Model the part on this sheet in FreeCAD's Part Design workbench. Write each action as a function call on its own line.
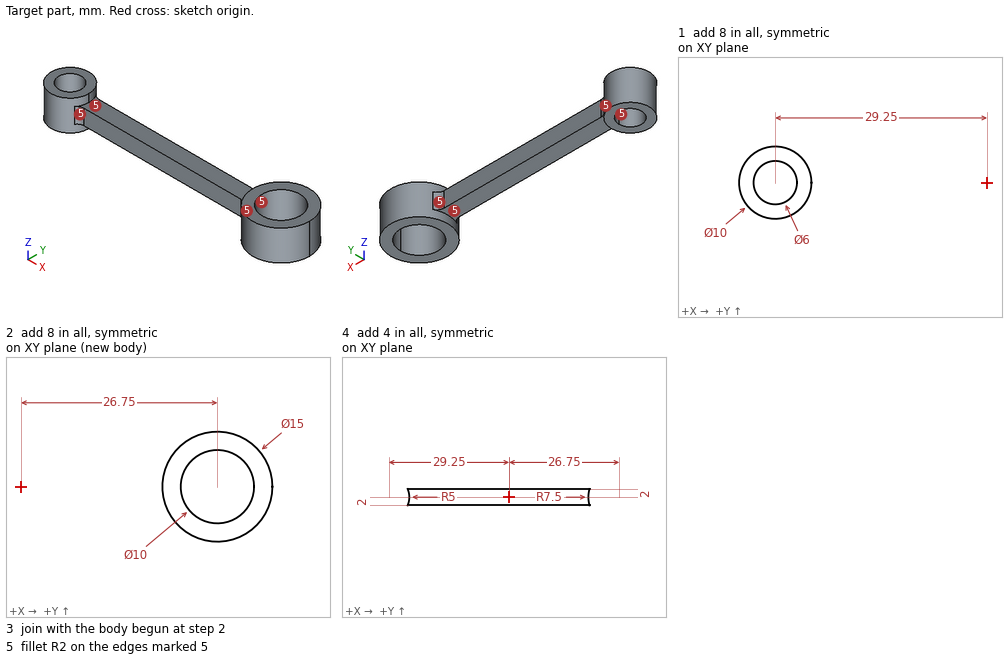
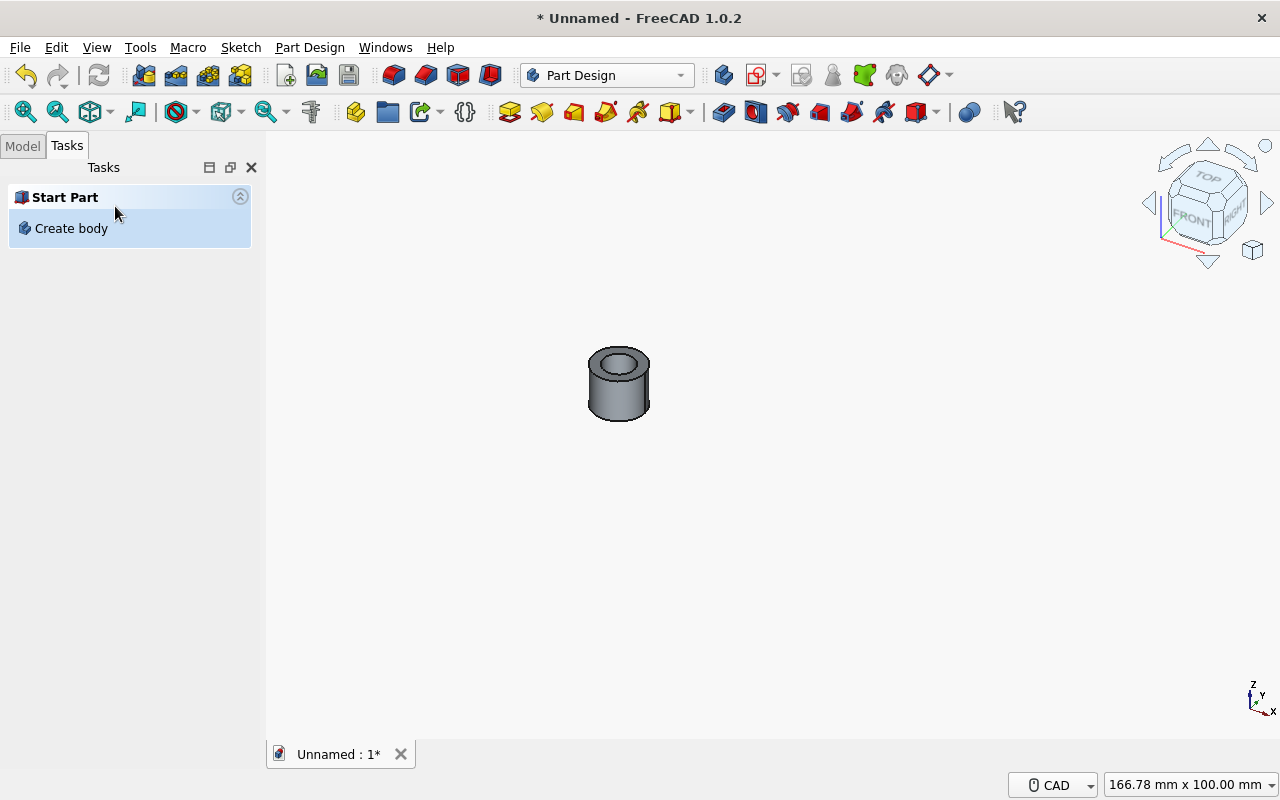
click(26, 112)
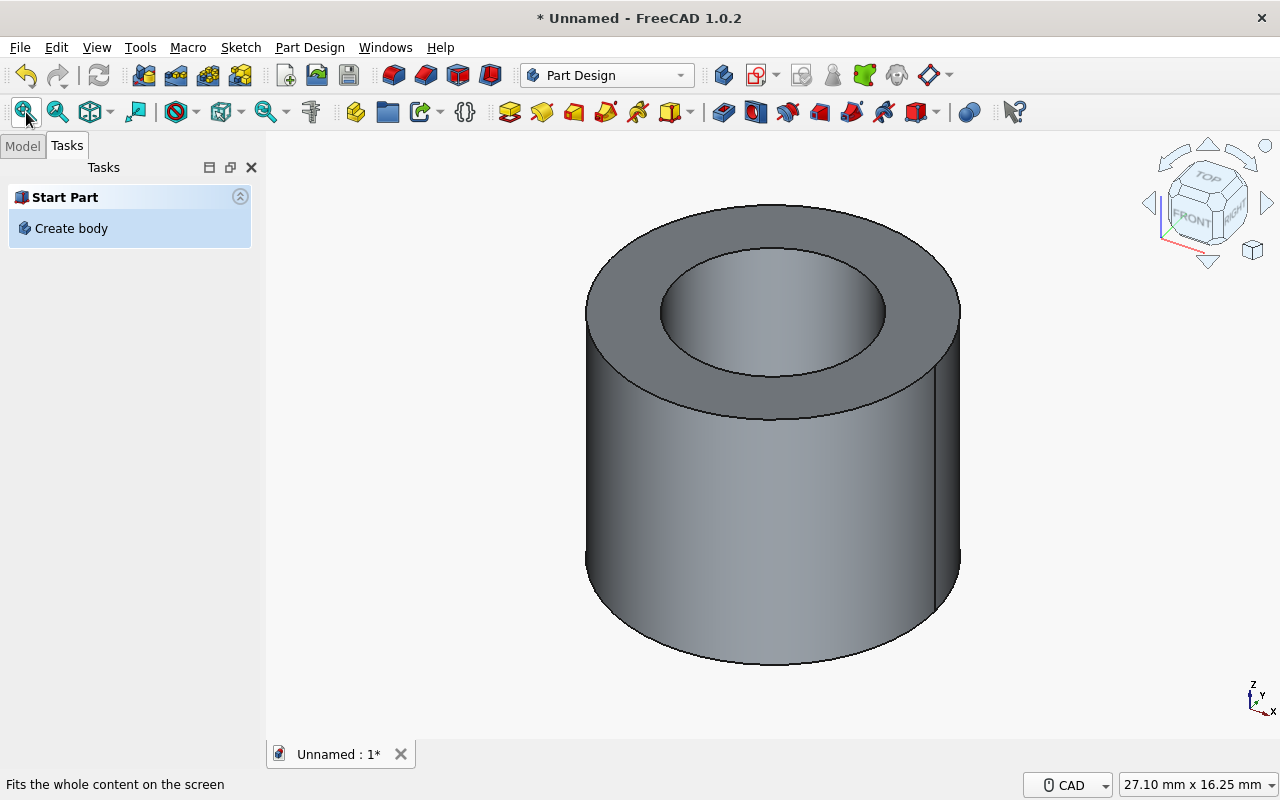
click(724, 76)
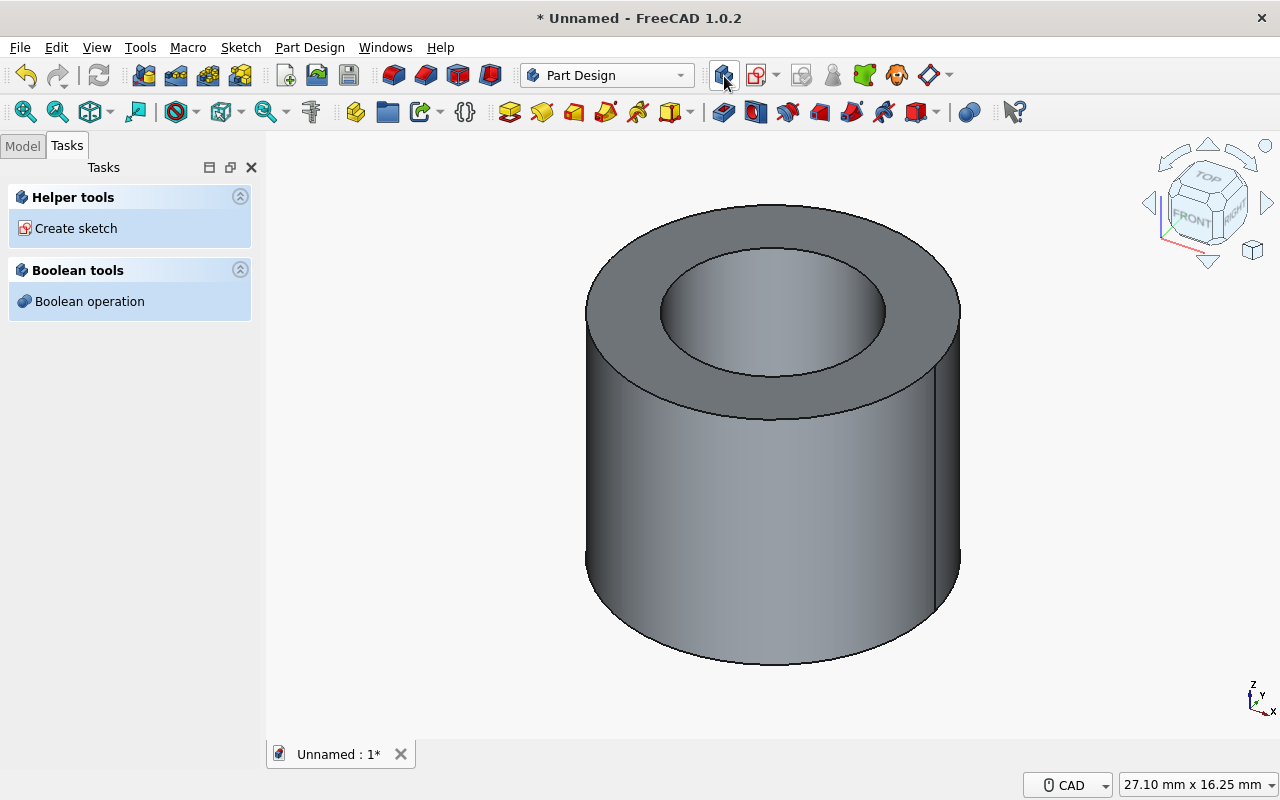
click(306, 699)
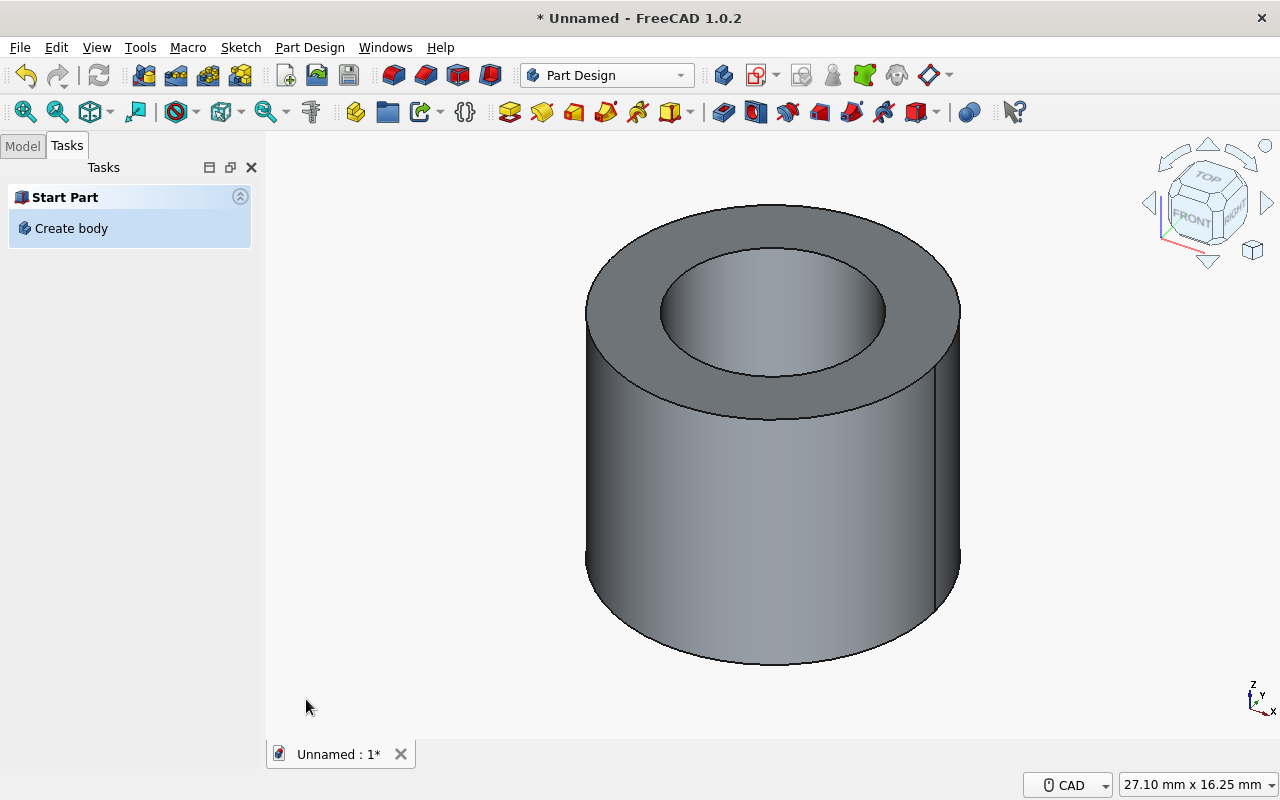
click(756, 76)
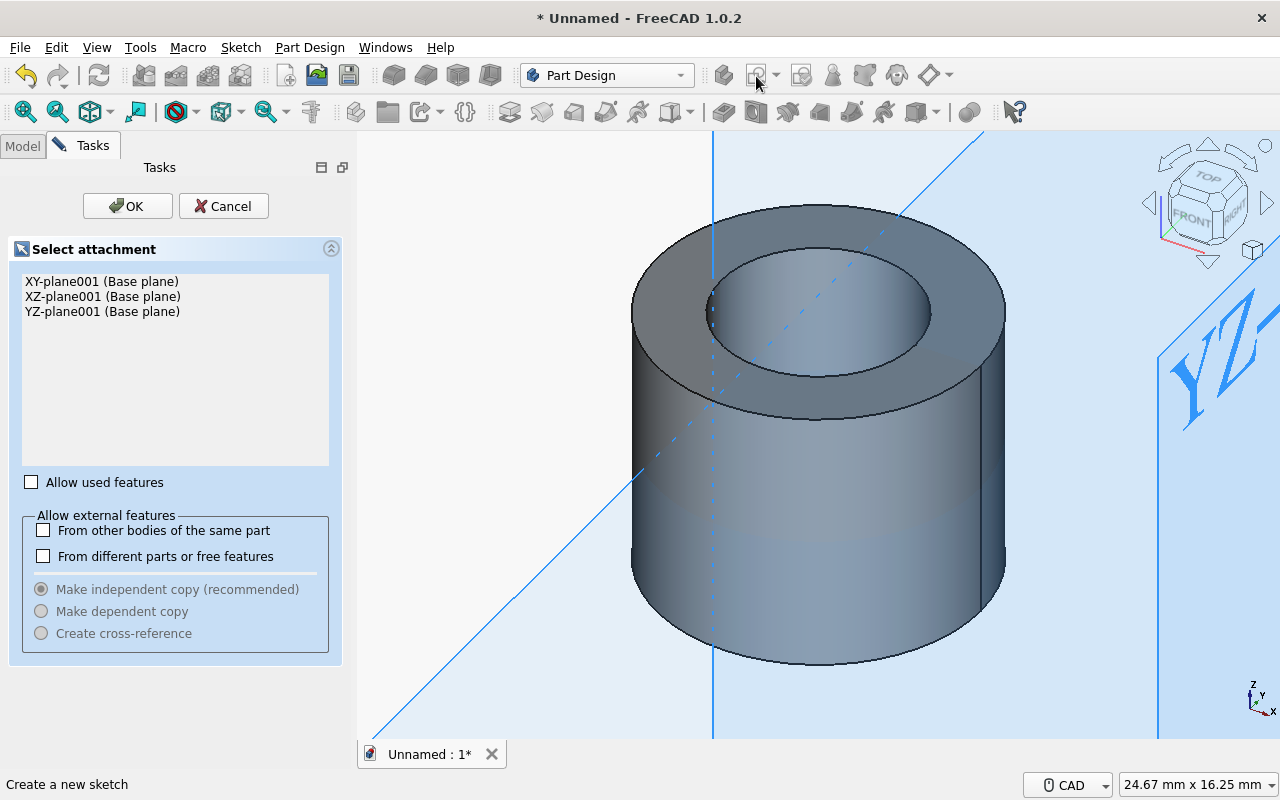
click(82, 282)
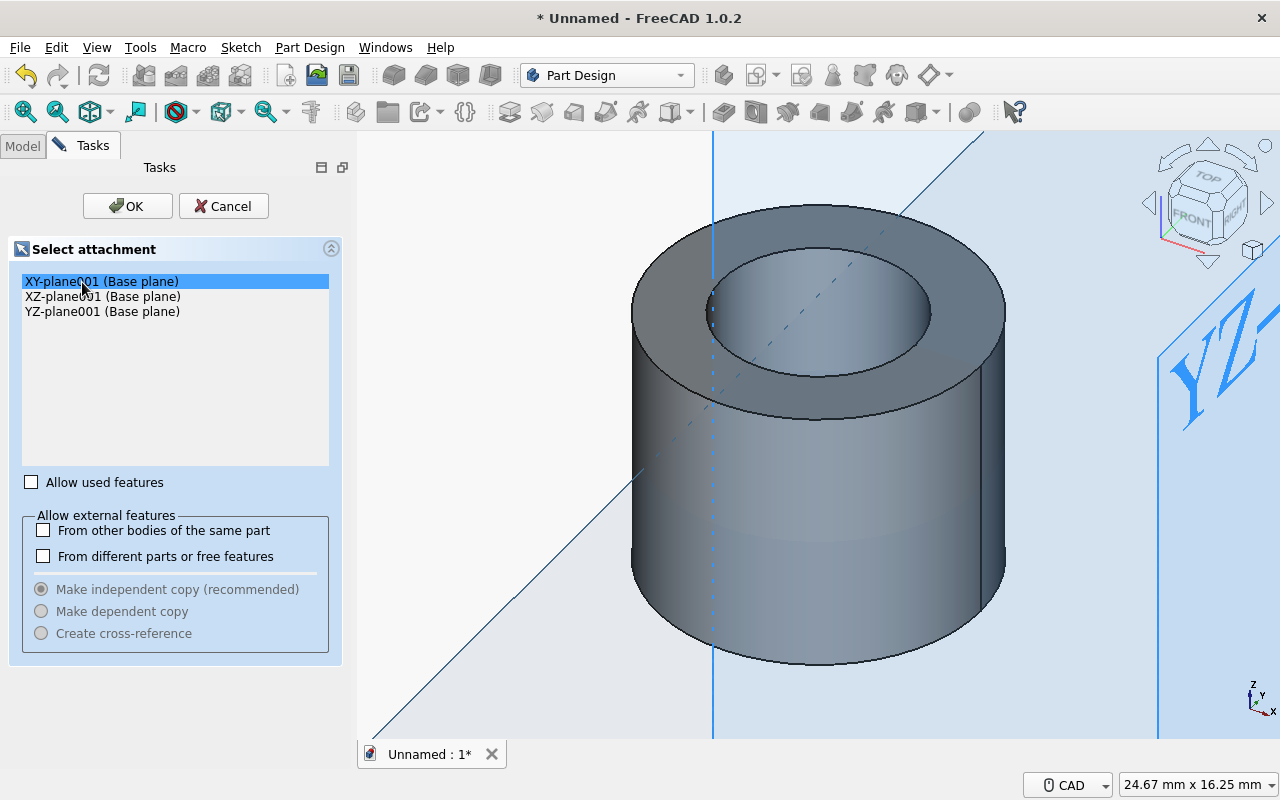
click(128, 206)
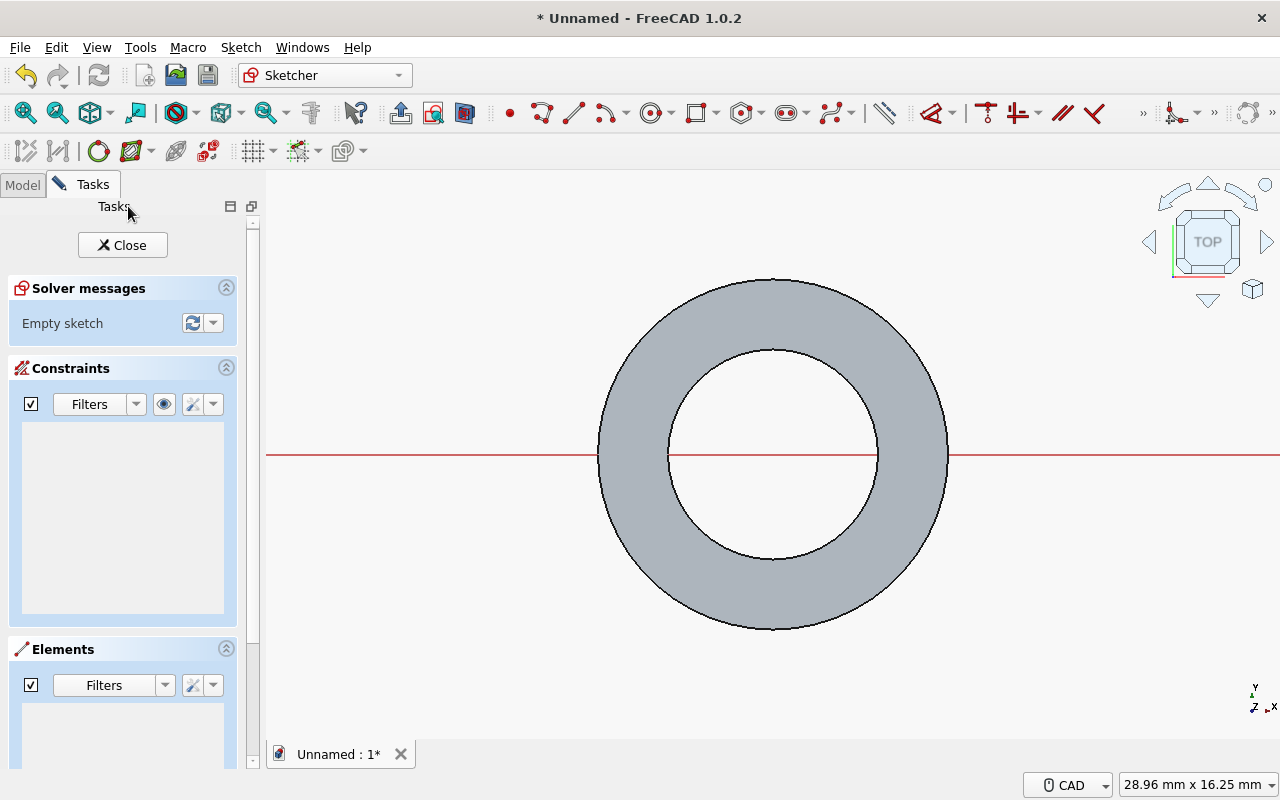
scroll(294, 454, down, 7)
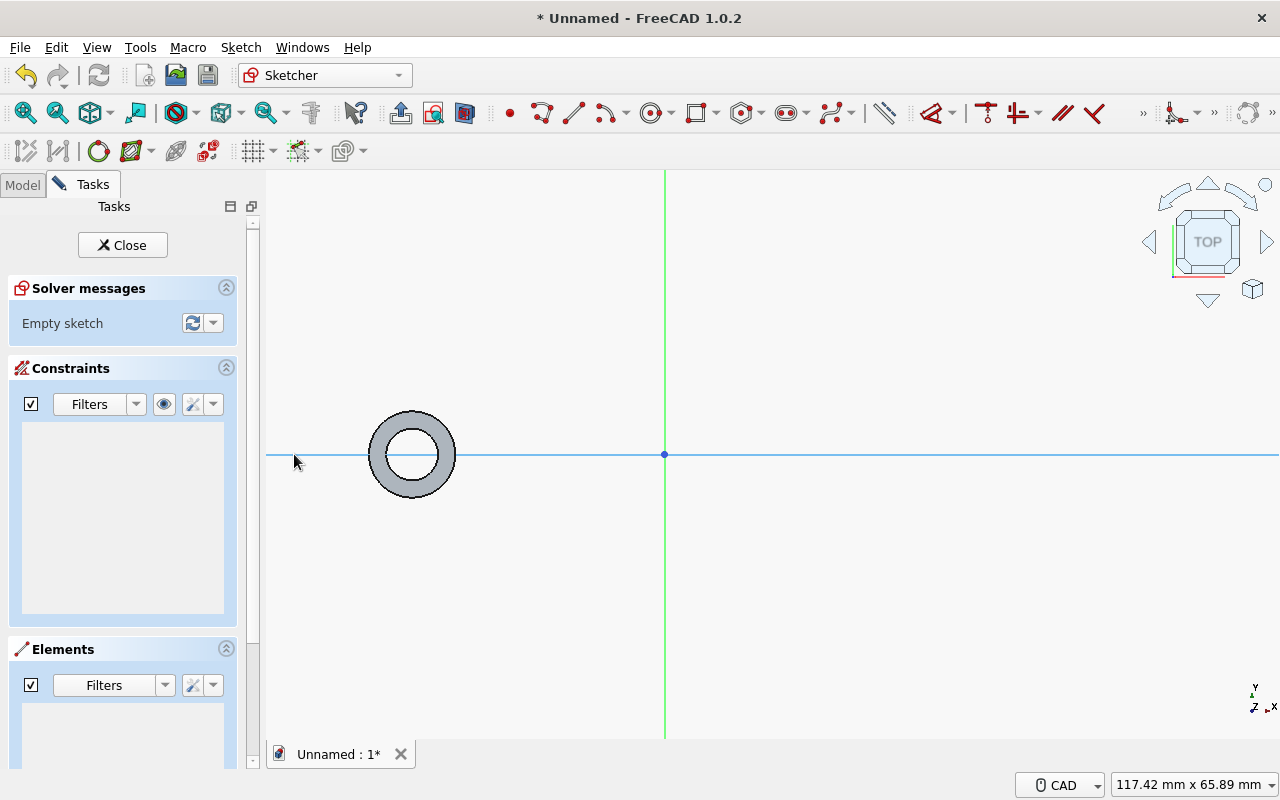
scroll(944, 454, up, 3)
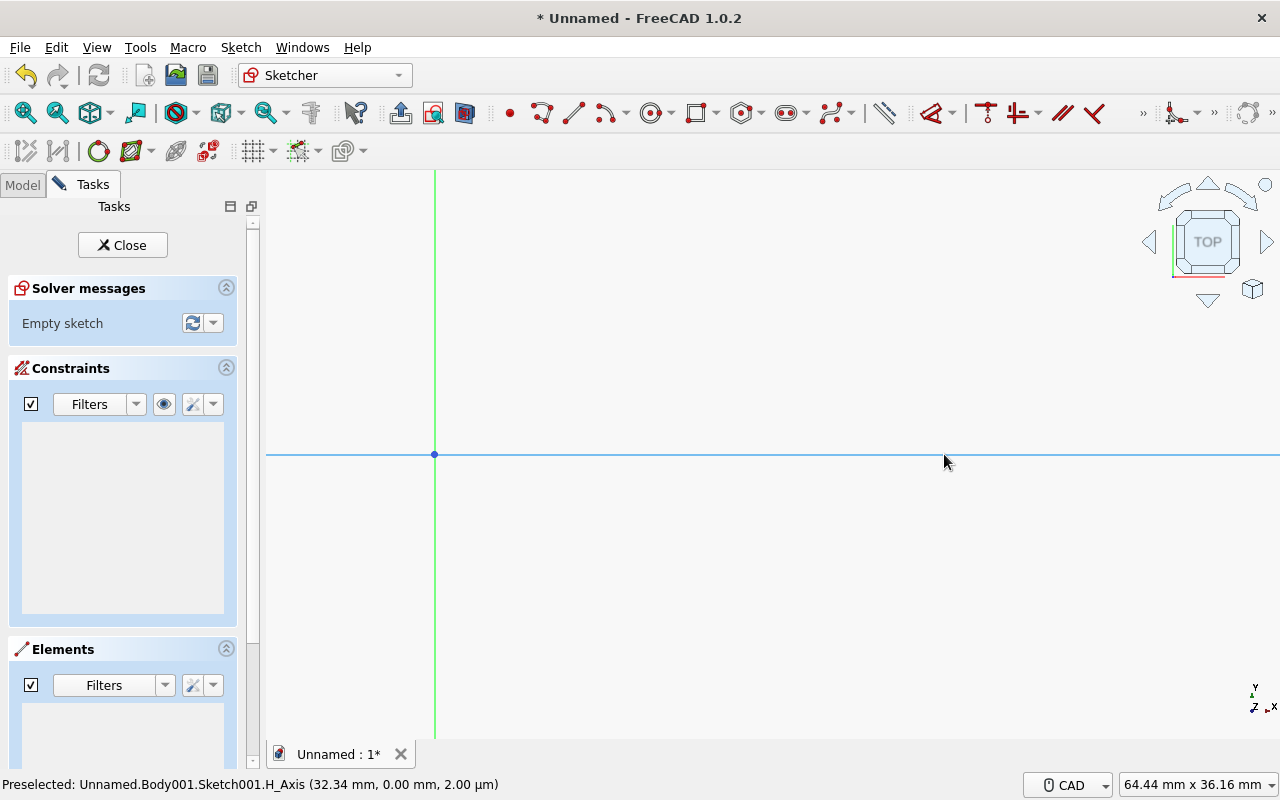
key(g)
key(c)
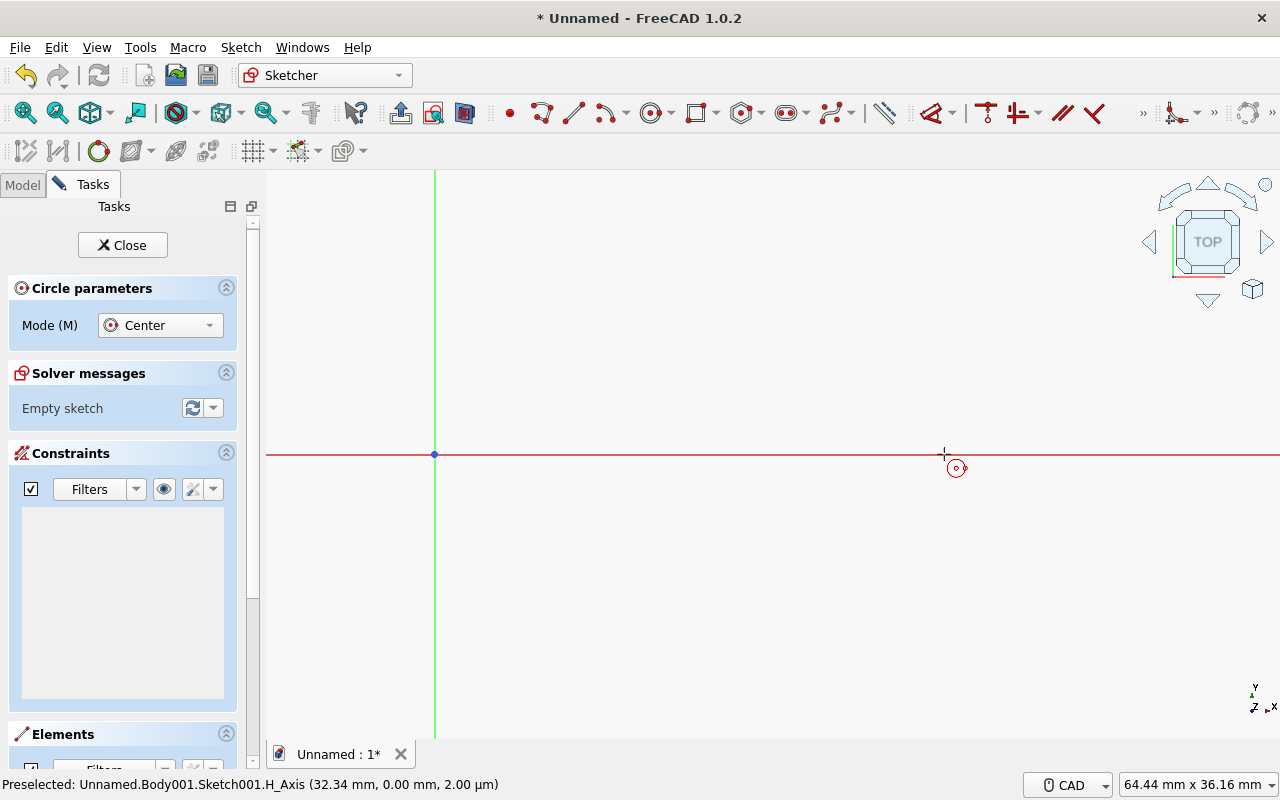
click(856, 454)
click(939, 371)